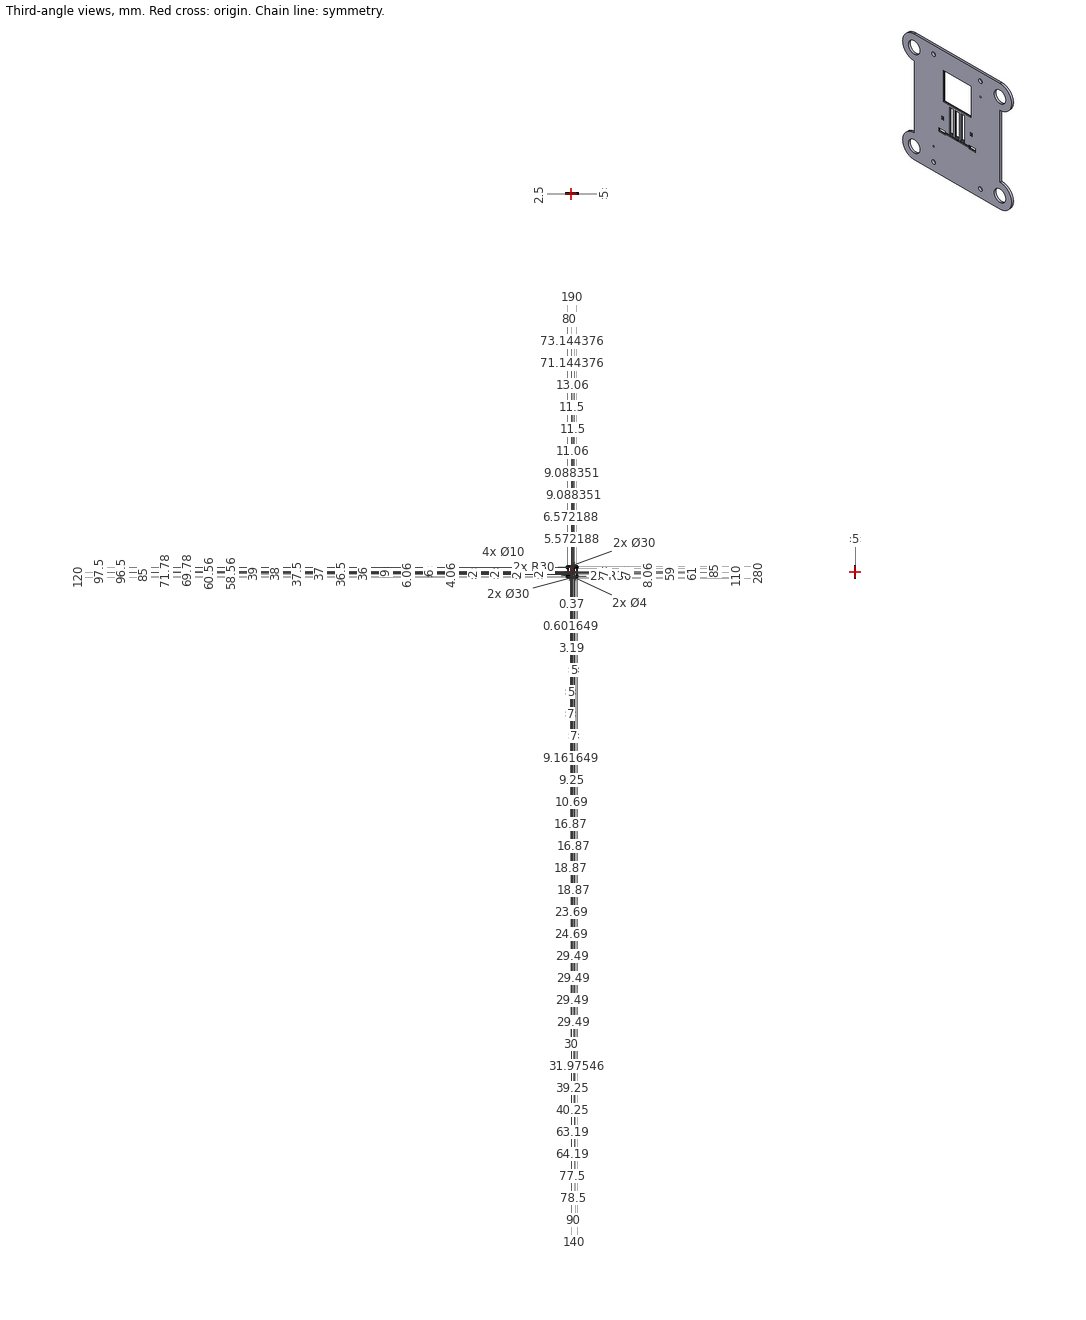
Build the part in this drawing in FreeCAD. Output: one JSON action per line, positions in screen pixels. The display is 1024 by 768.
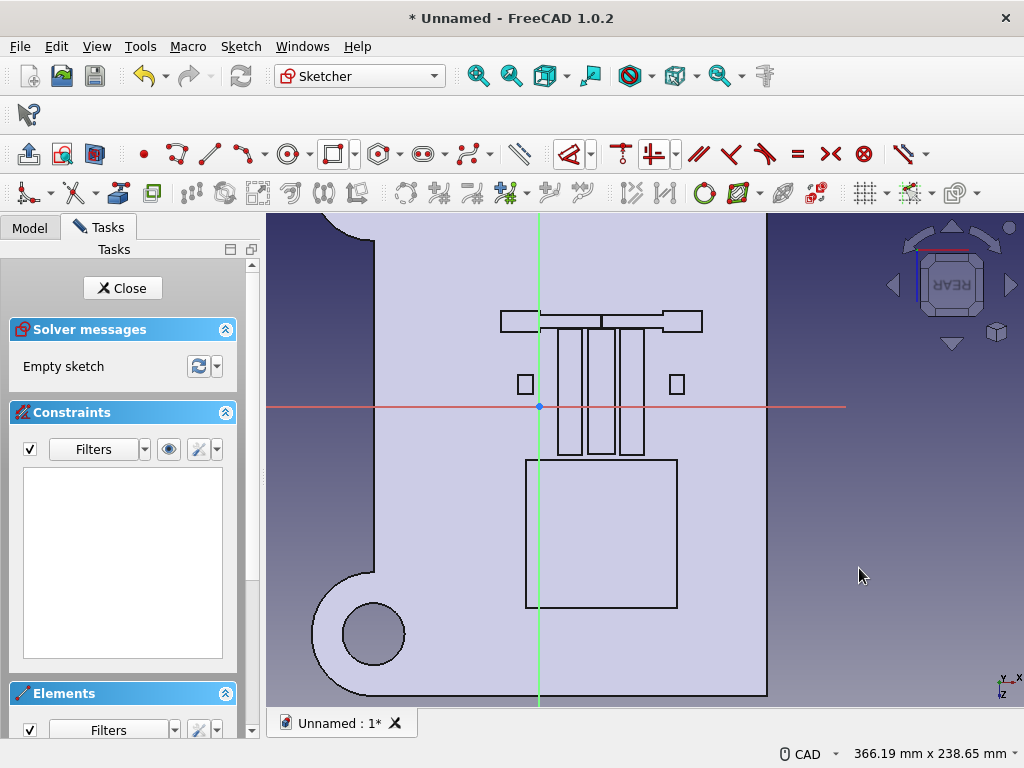
{"action": "left_click", "coordinate": [332, 154]}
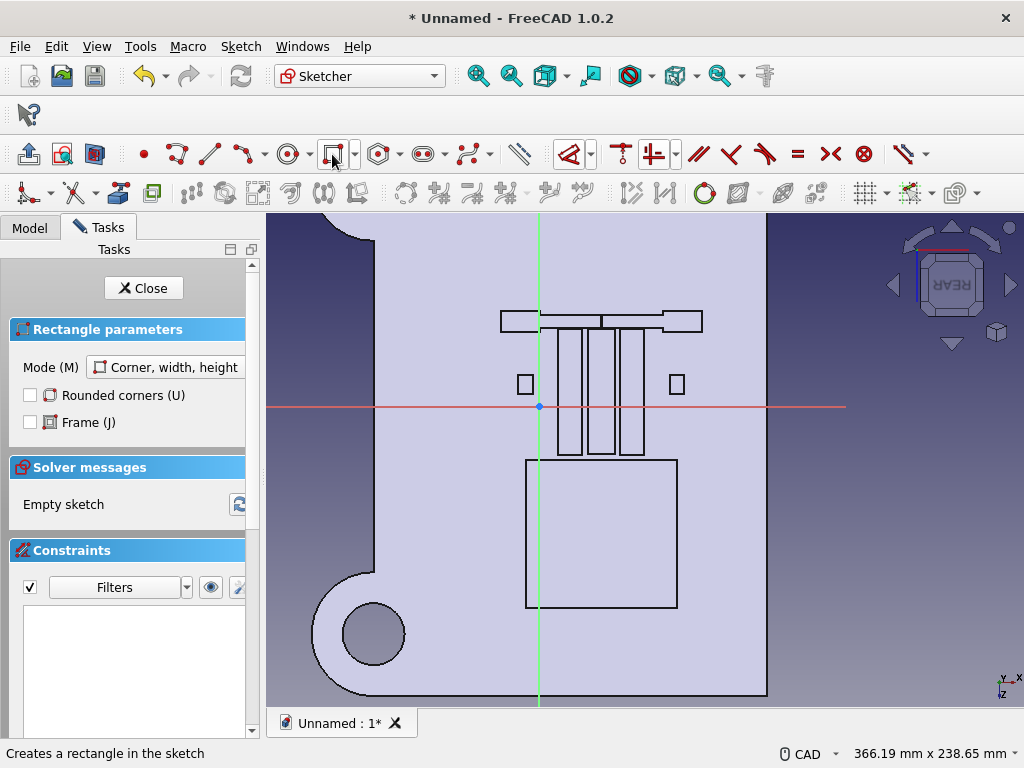
{"action": "left_click", "coordinate": [590, 331]}
{"action": "left_click", "coordinate": [613, 452]}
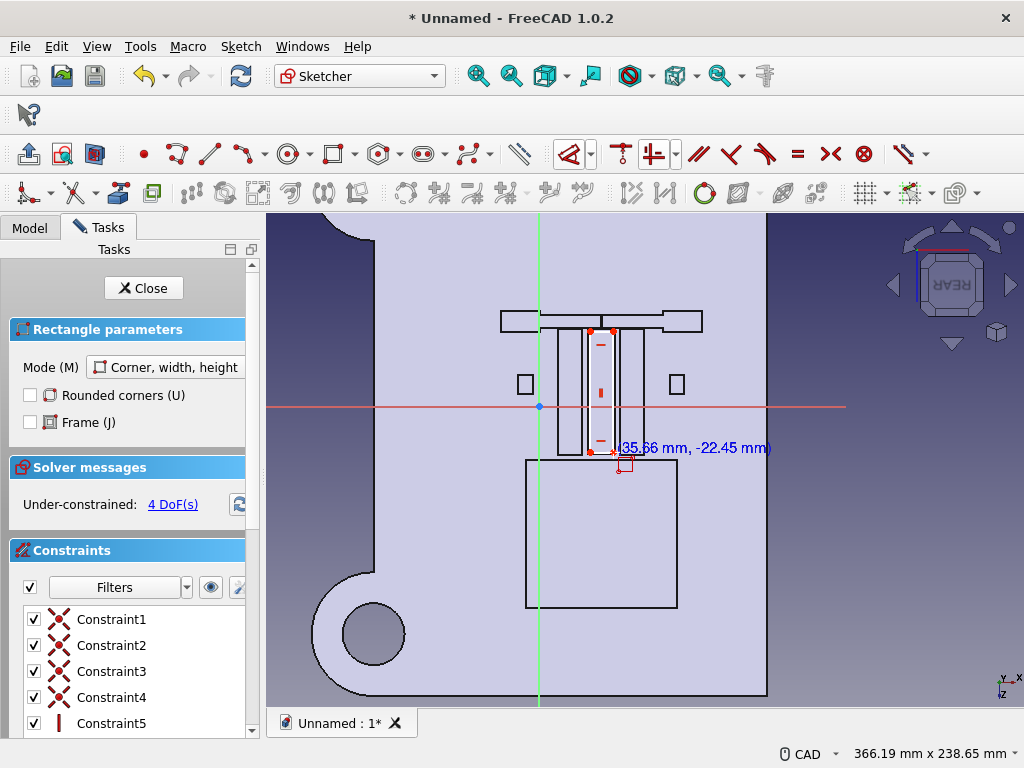
{"action": "left_click", "coordinate": [177, 154]}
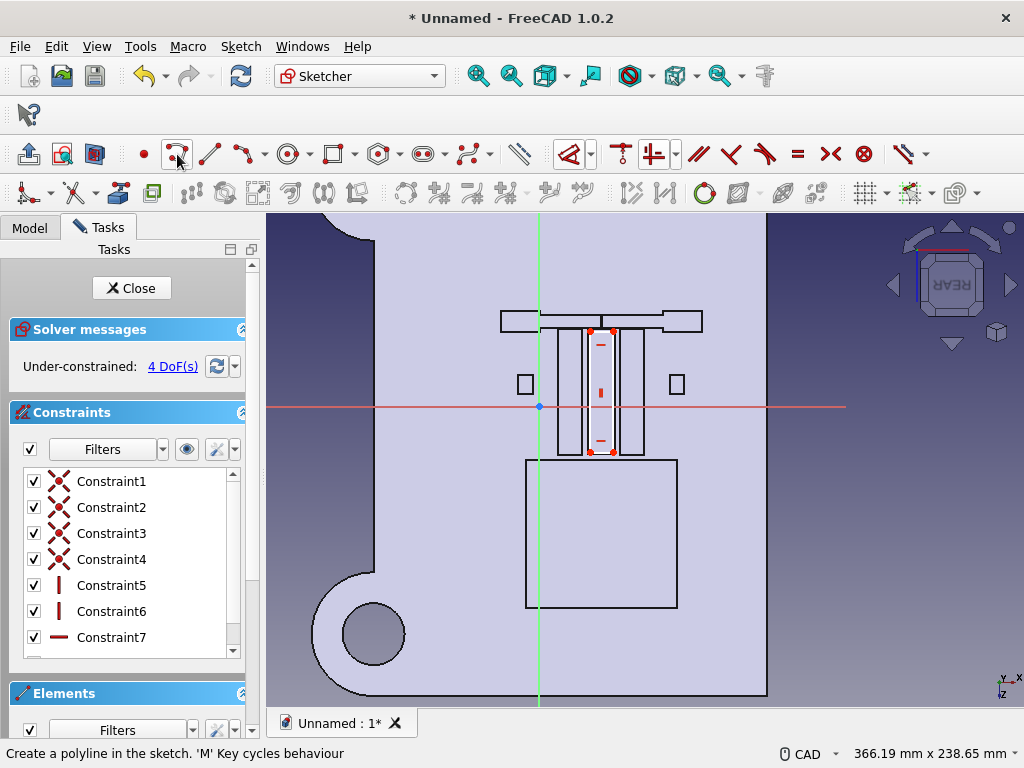
{"action": "scroll", "coordinate": [538, 330], "scroll_direction": "up", "scroll_amount": 13}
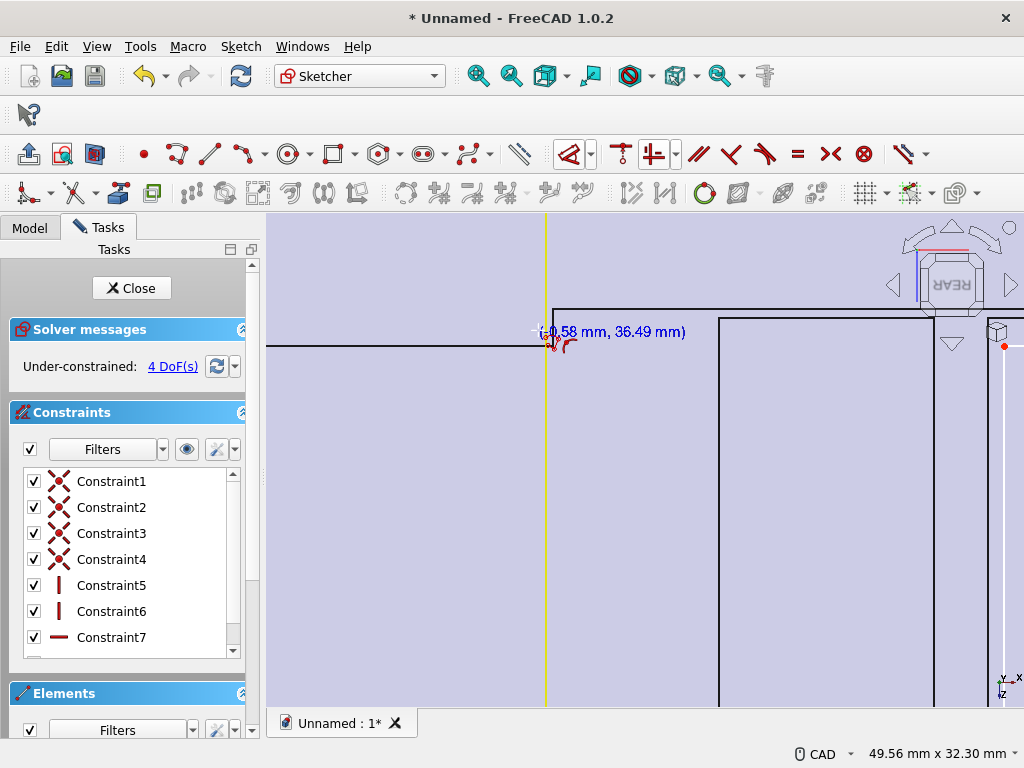
{"action": "left_click", "coordinate": [533, 326]}
{"action": "left_click", "coordinate": [533, 270]}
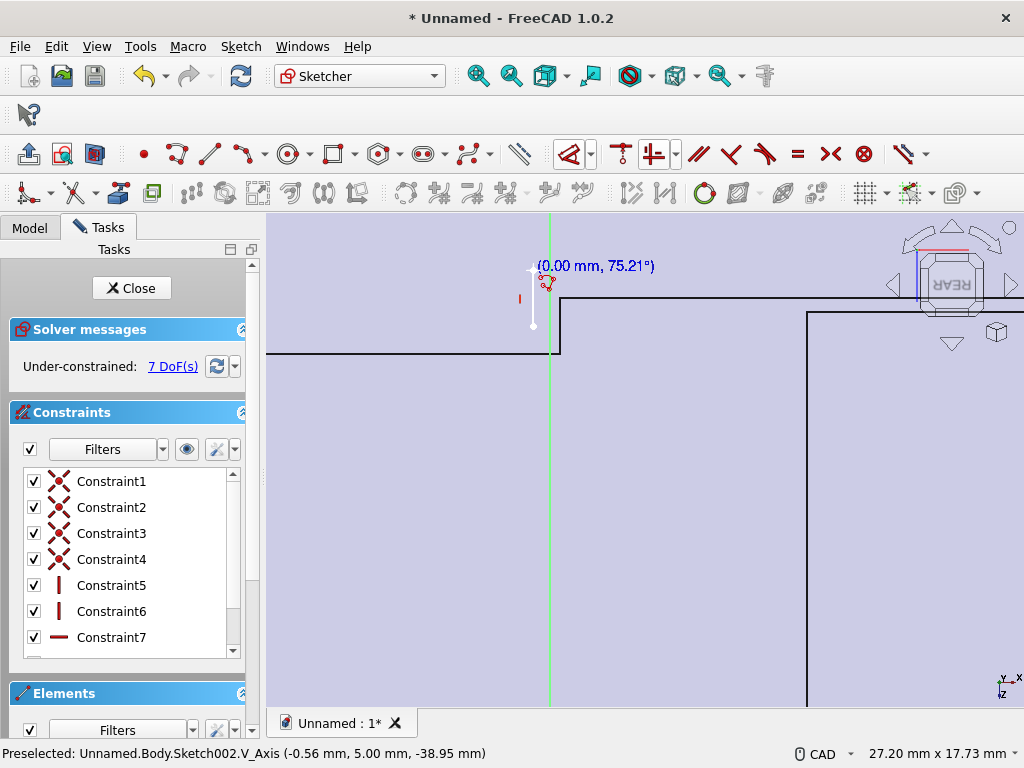
{"action": "scroll", "coordinate": [512, 330], "scroll_direction": "down", "scroll_amount": 13}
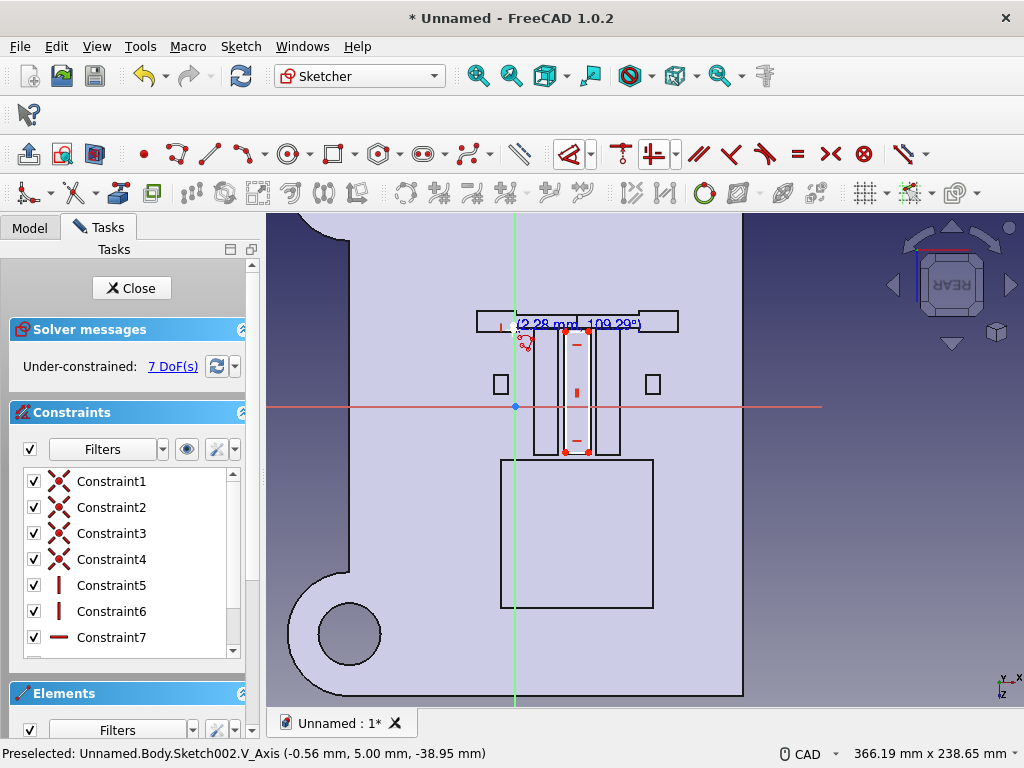
{"action": "scroll", "coordinate": [575, 326], "scroll_direction": "up", "scroll_amount": 6}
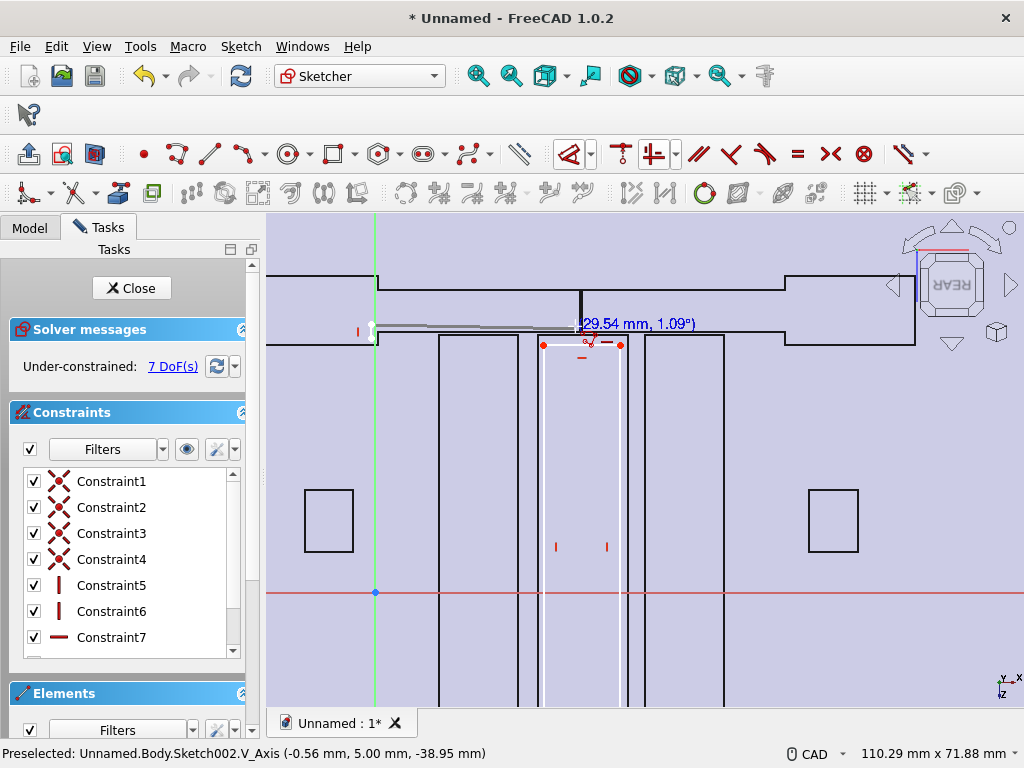
{"action": "left_click", "coordinate": [574, 325]}
{"action": "left_click", "coordinate": [574, 297]}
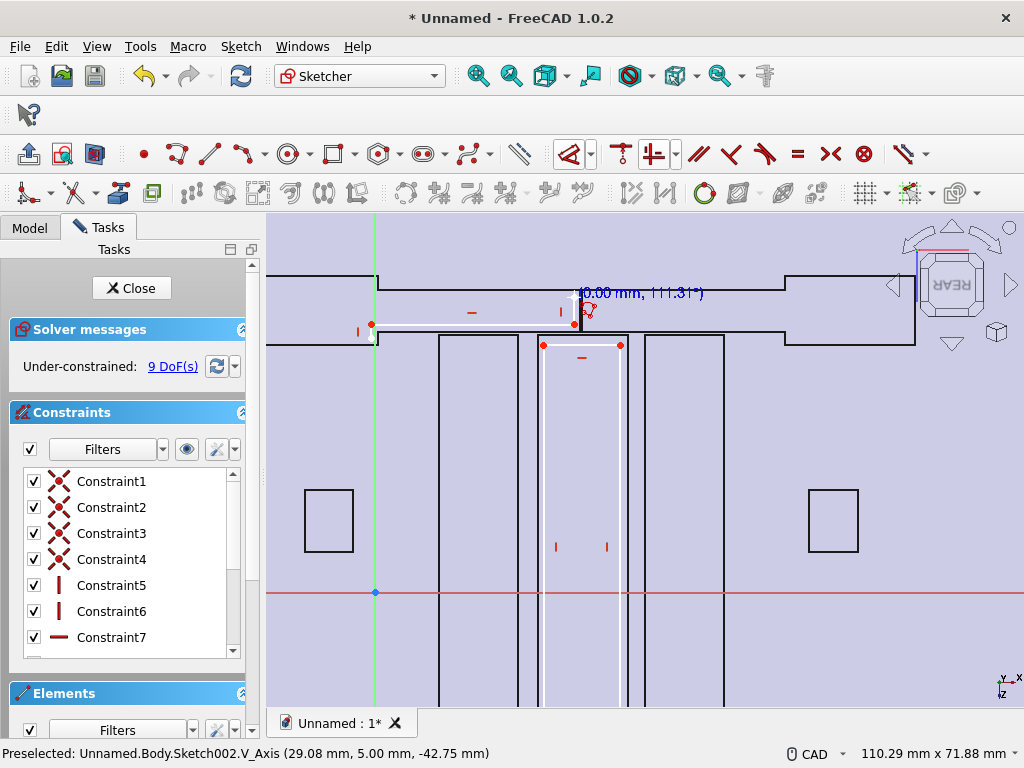
{"action": "scroll", "coordinate": [371, 297], "scroll_direction": "up", "scroll_amount": 7}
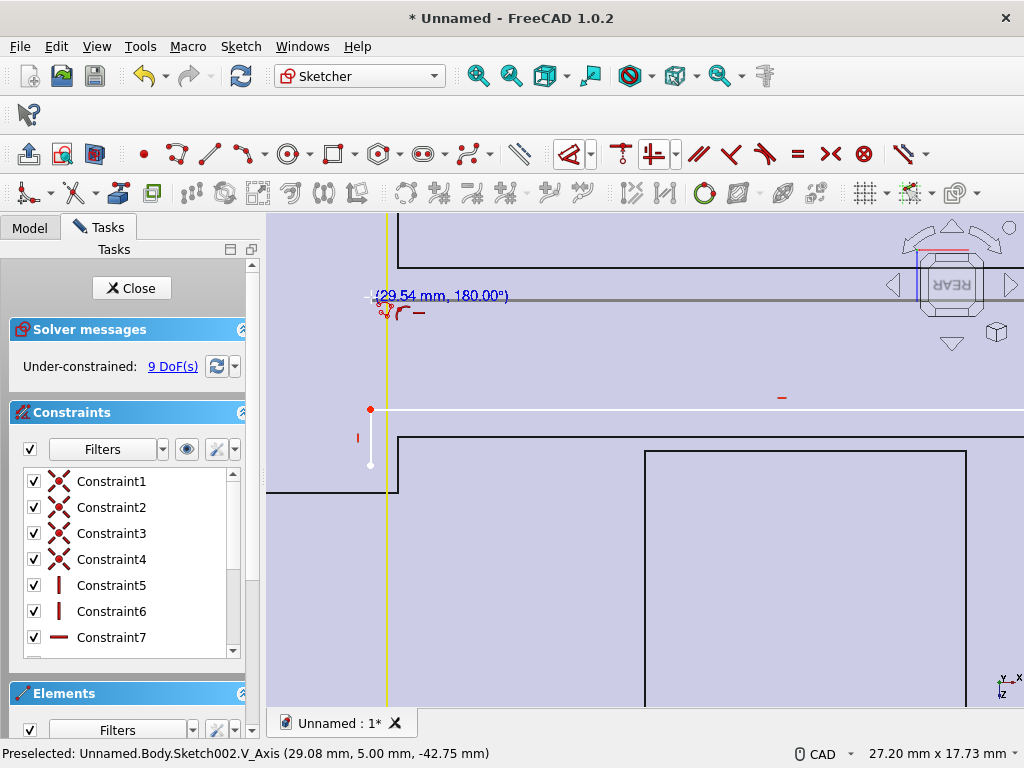
{"action": "left_click", "coordinate": [371, 296]}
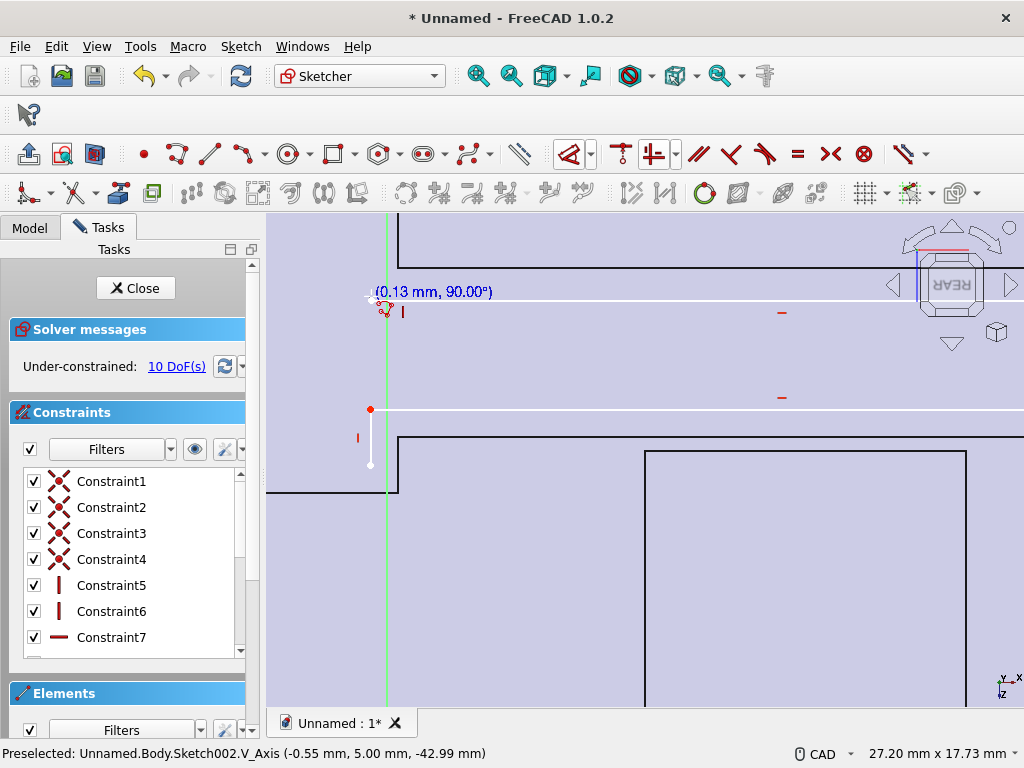
{"action": "scroll", "coordinate": [525, 319], "scroll_direction": "down", "scroll_amount": 13}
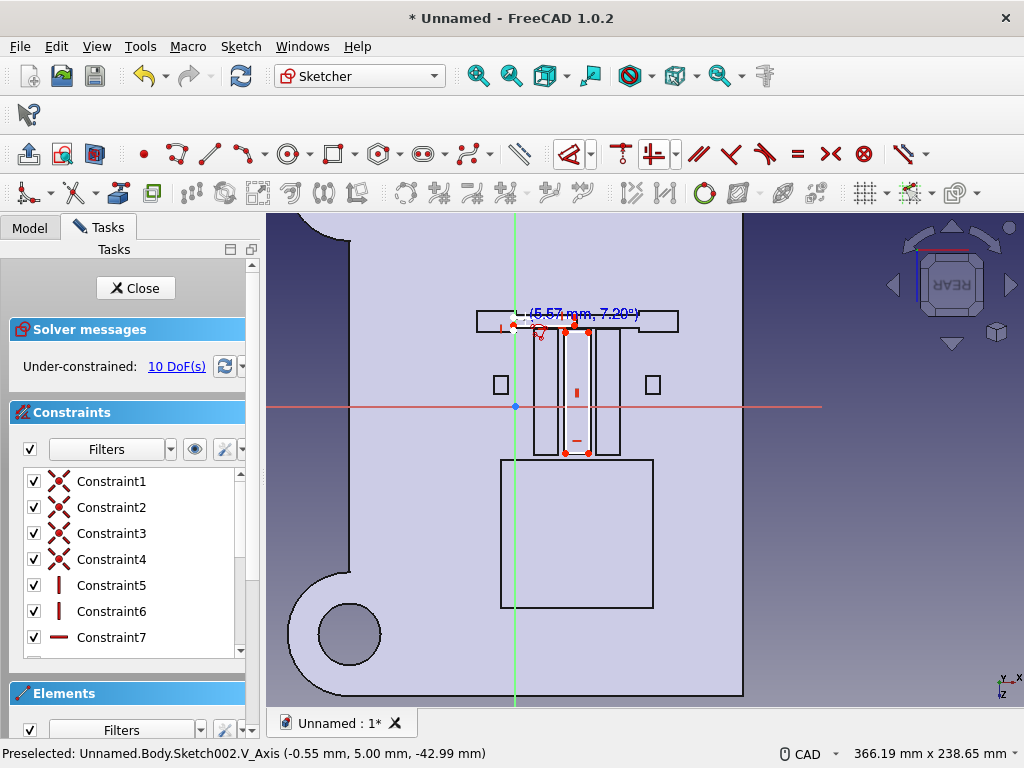
{"action": "scroll", "coordinate": [514, 313], "scroll_direction": "up", "scroll_amount": 13}